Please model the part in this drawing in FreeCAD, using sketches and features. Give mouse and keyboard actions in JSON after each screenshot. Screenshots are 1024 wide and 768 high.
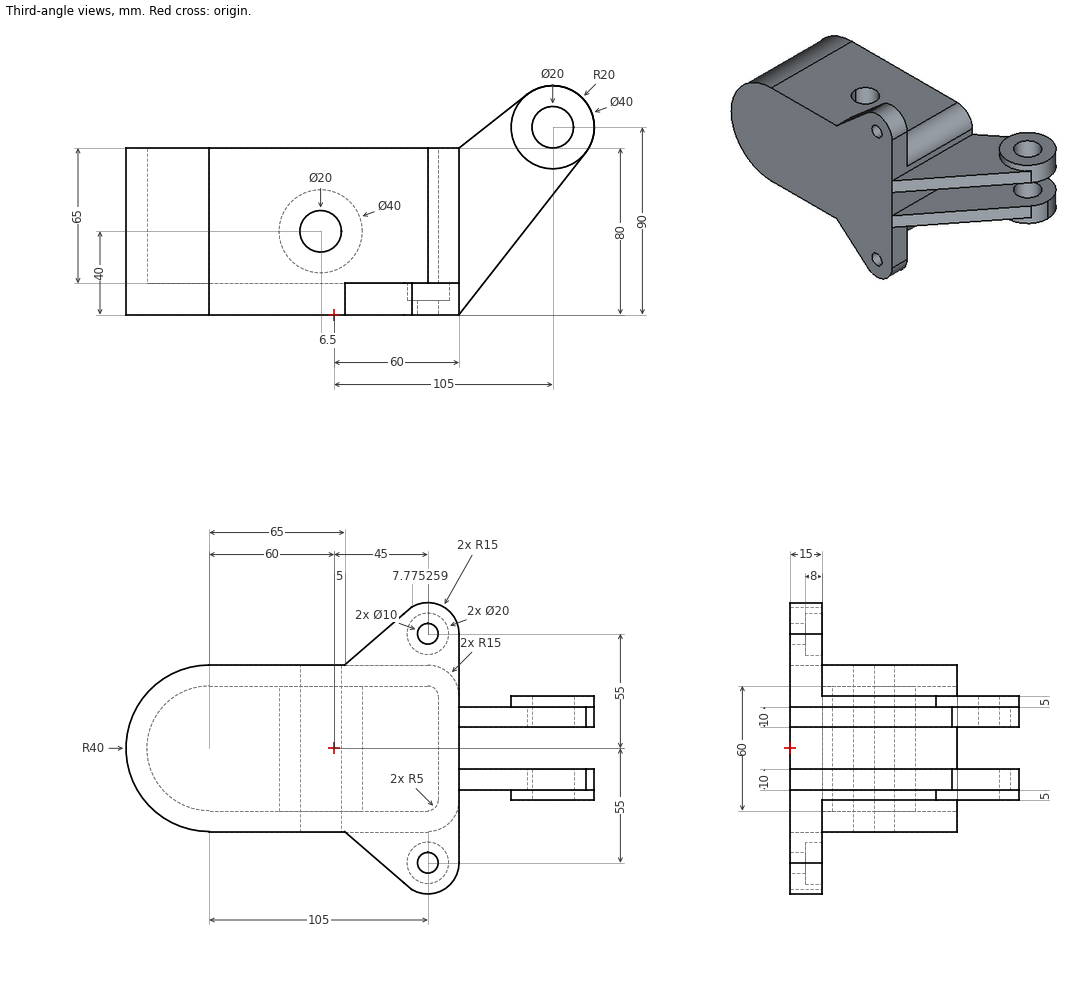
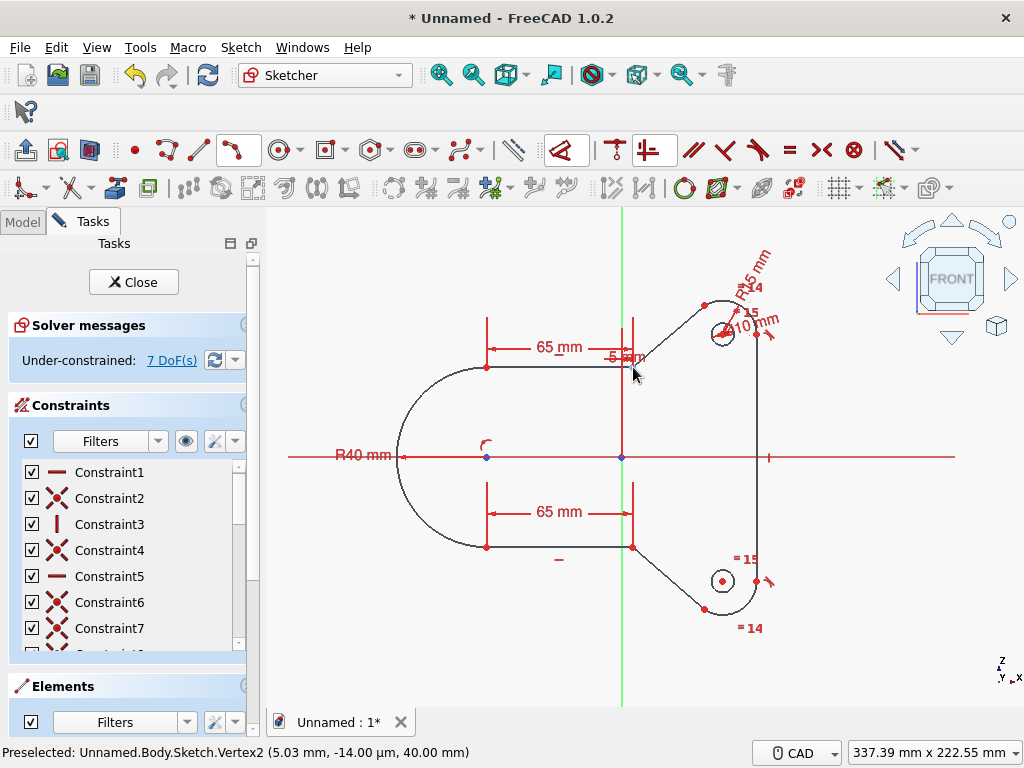
{"action": "scroll", "coordinate": [633, 547], "scroll_direction": "up", "scroll_amount": 7}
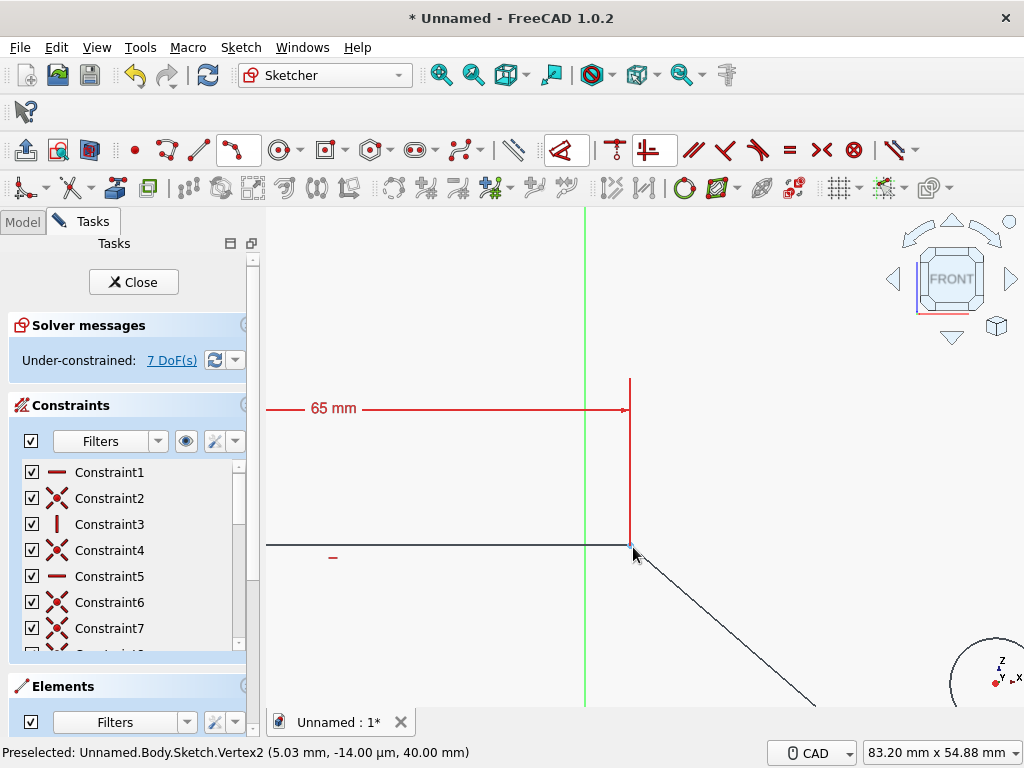
{"action": "left_click", "coordinate": [630, 545]}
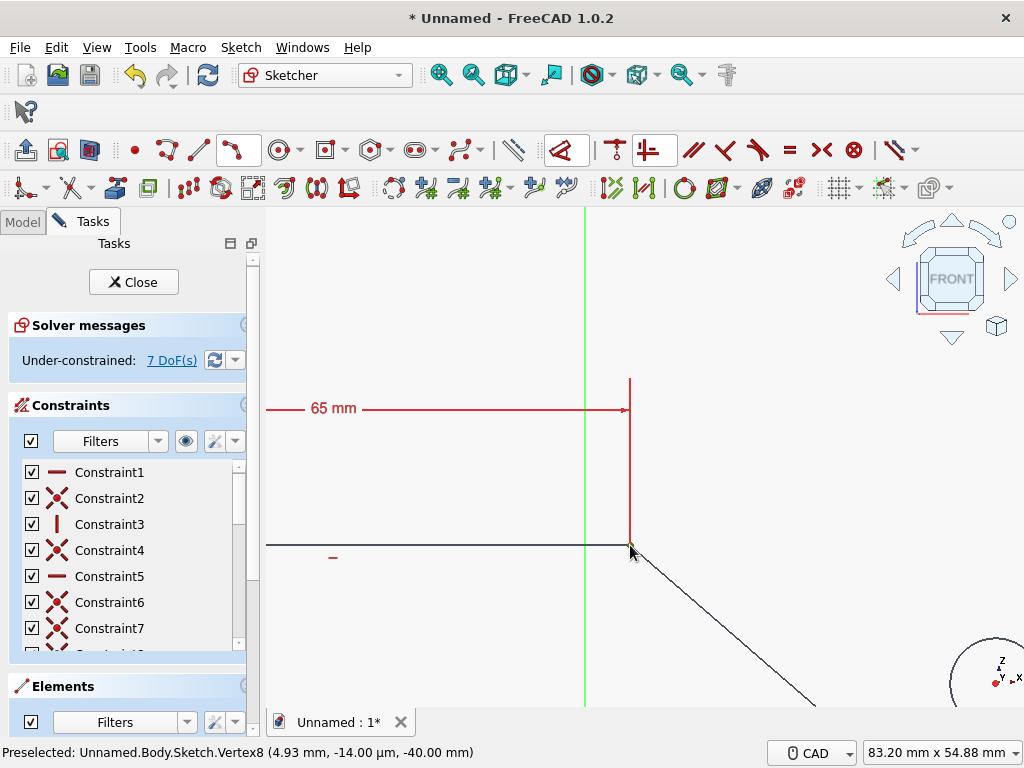
{"action": "key", "text": "l"}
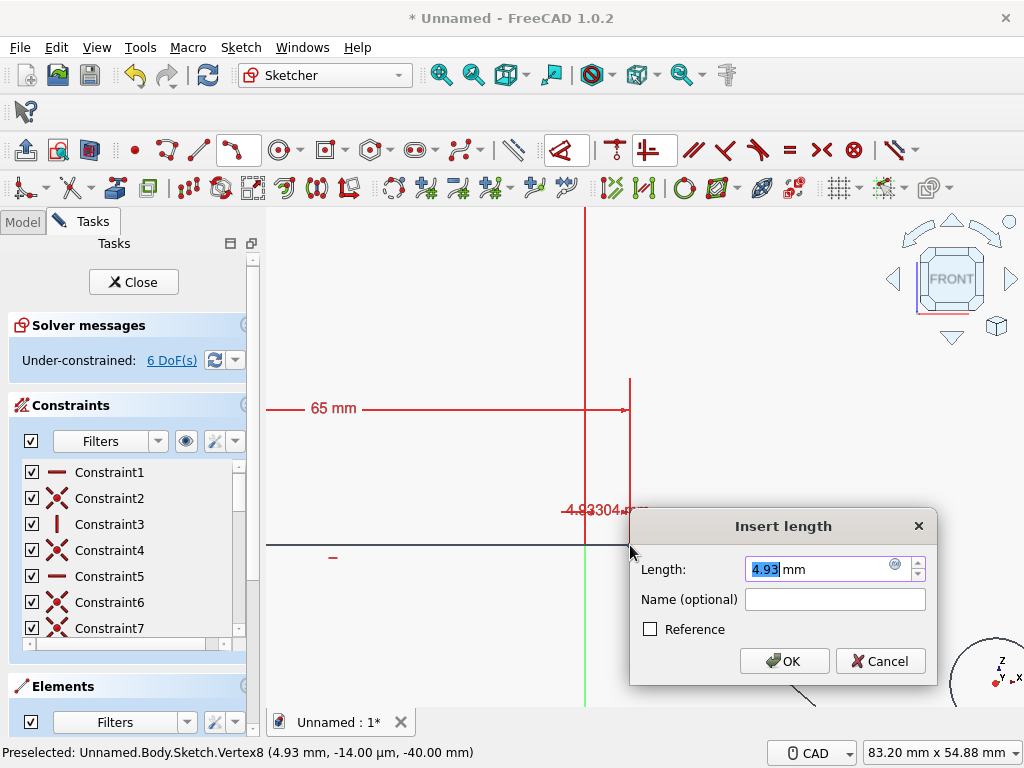
{"action": "type", "text": "5"}
{"action": "key", "text": "Return"}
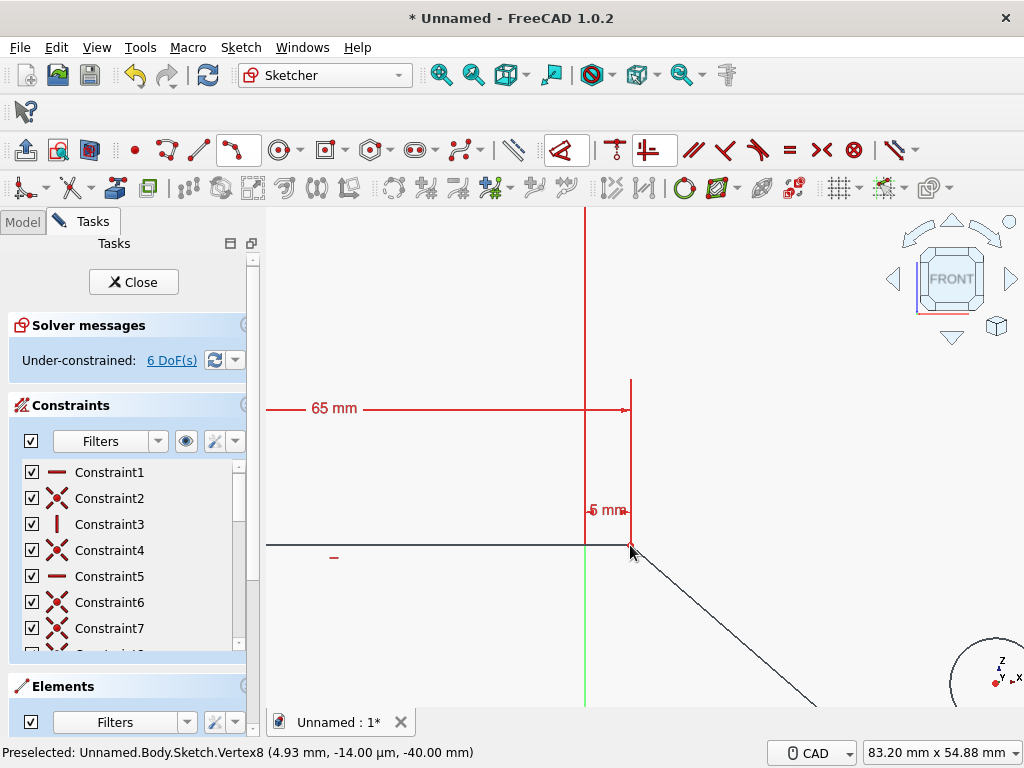
{"action": "scroll", "coordinate": [633, 547], "scroll_direction": "down", "scroll_amount": 7}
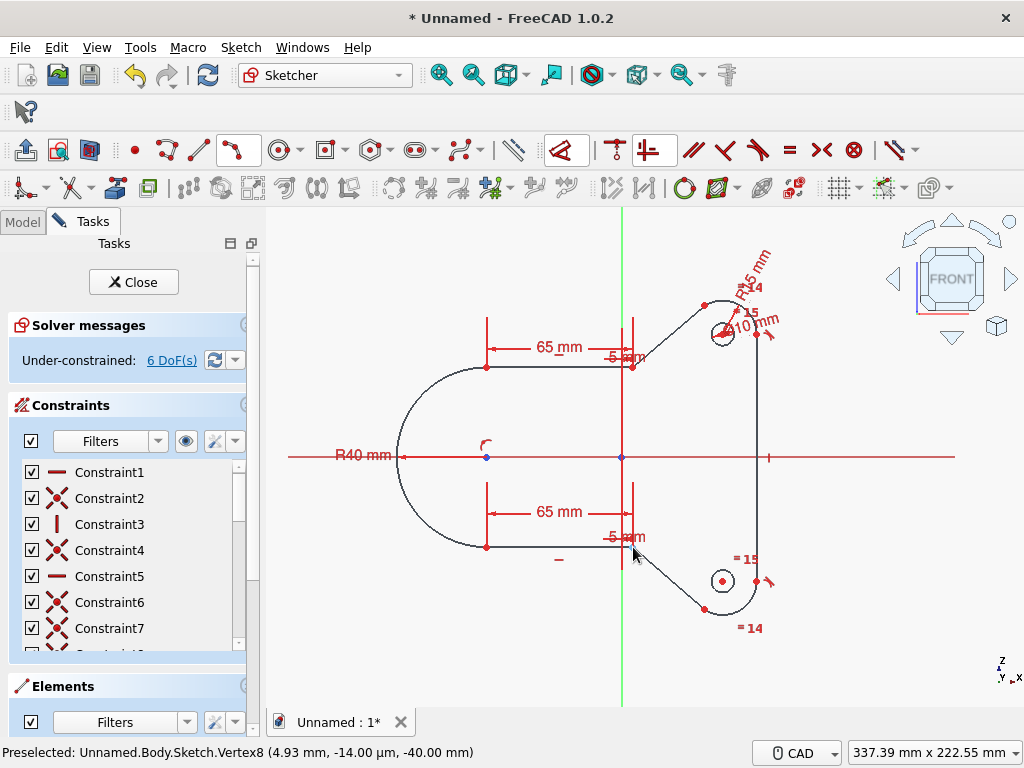
{"action": "left_click", "coordinate": [723, 334]}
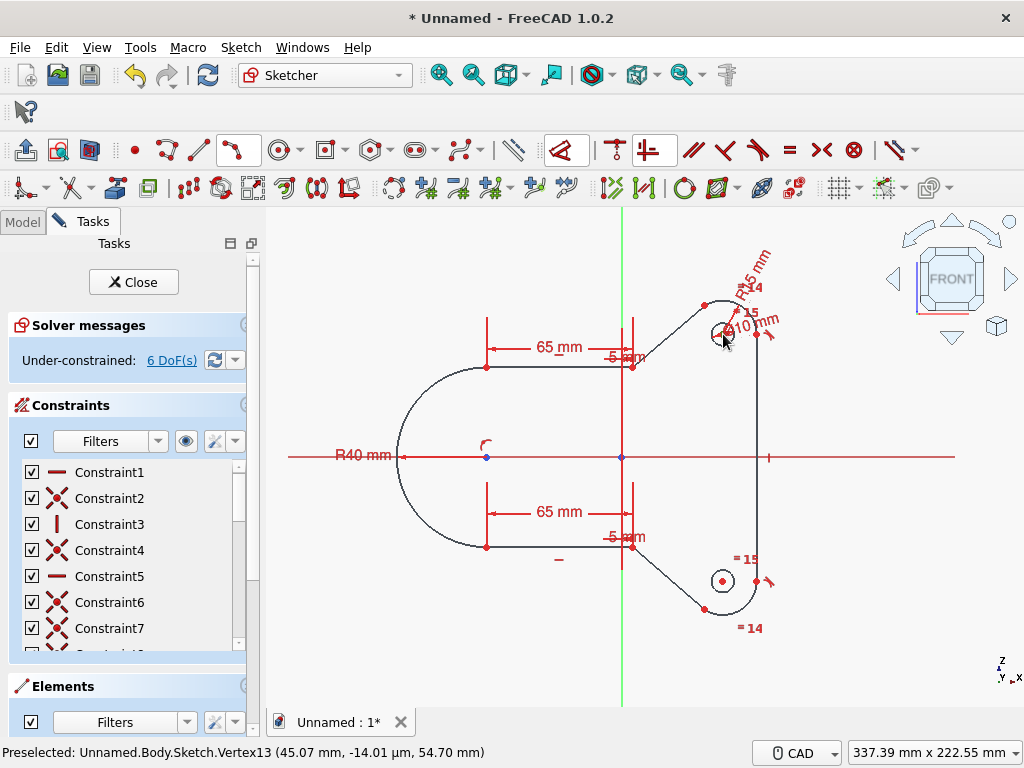
{"action": "left_click", "coordinate": [584, 150]}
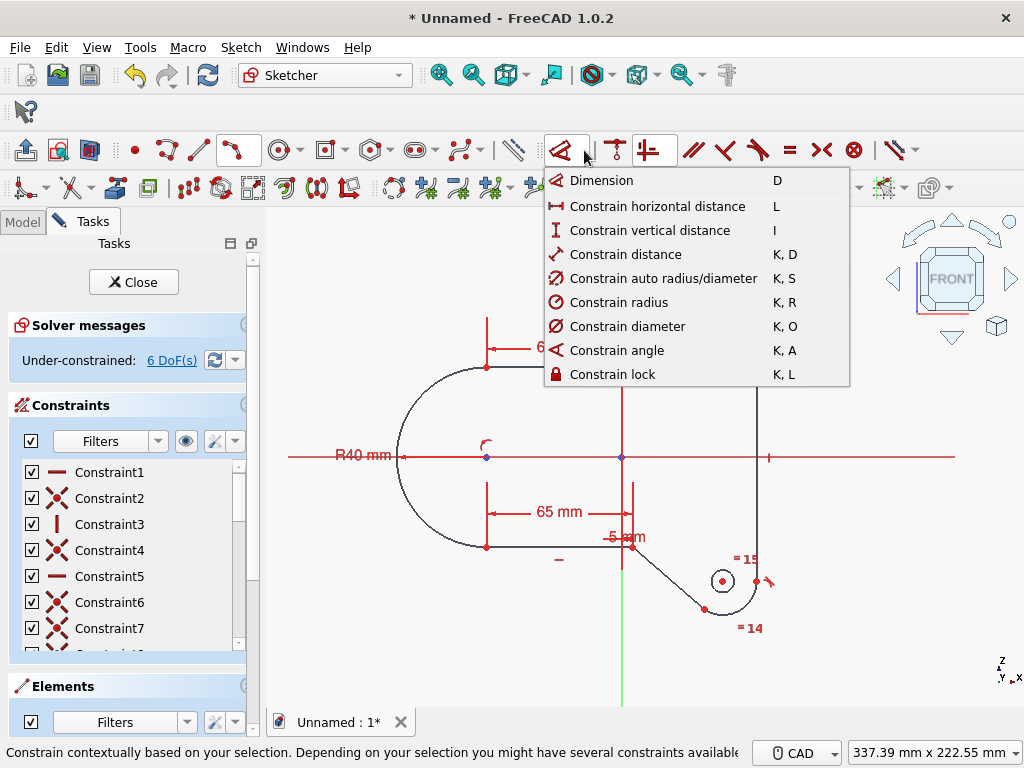
{"action": "left_click", "coordinate": [697, 206]}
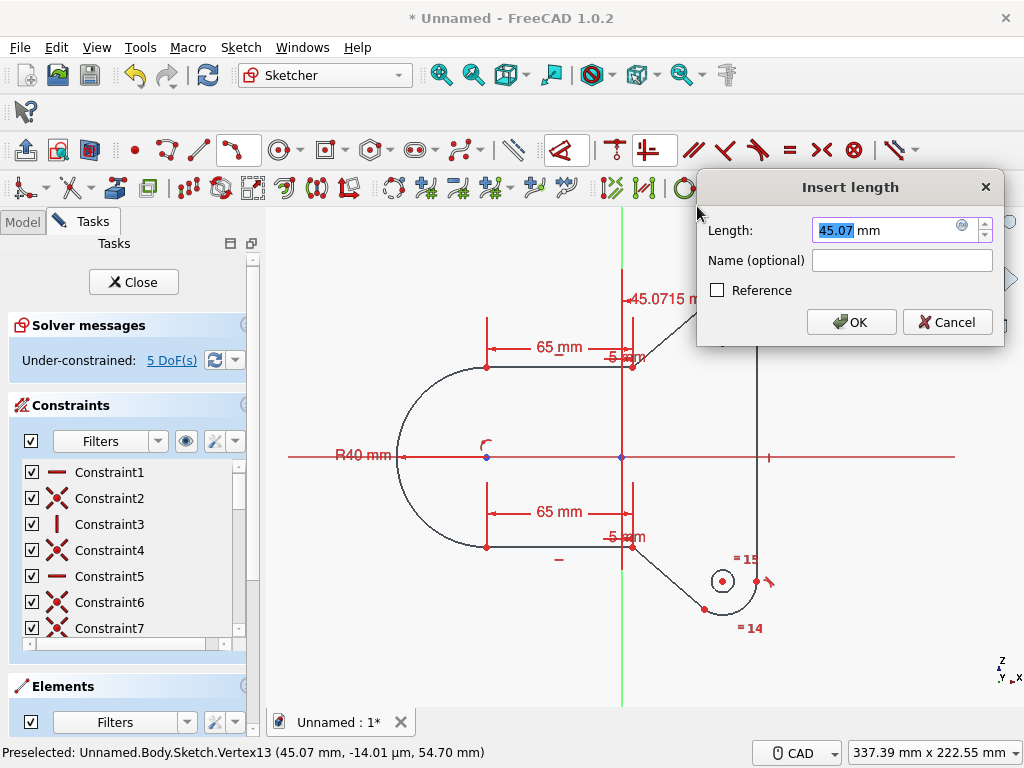
{"action": "type", "text": "45"}
{"action": "key", "text": "Return"}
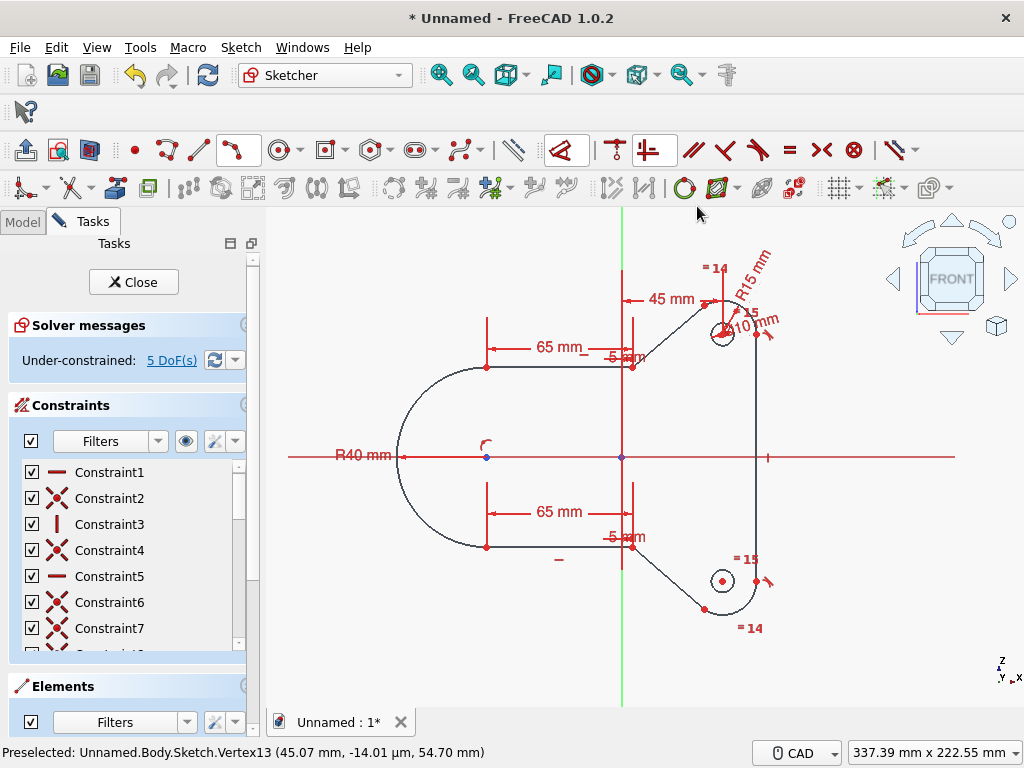
{"action": "left_click", "coordinate": [723, 334]}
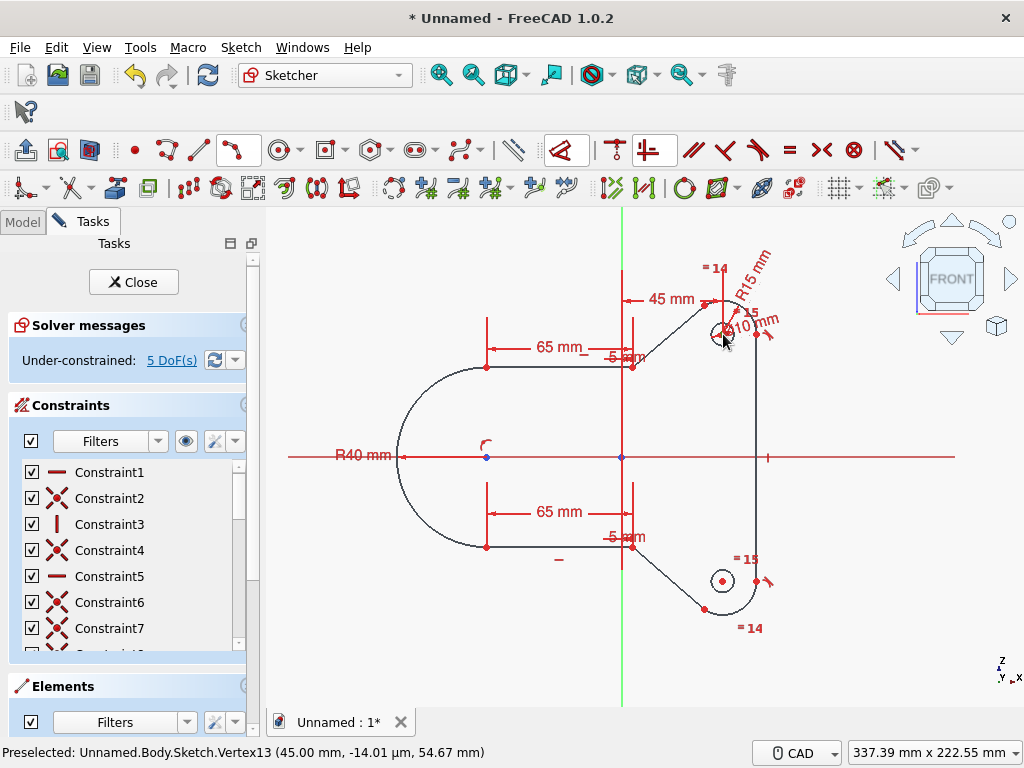
{"action": "left_click", "coordinate": [584, 150]}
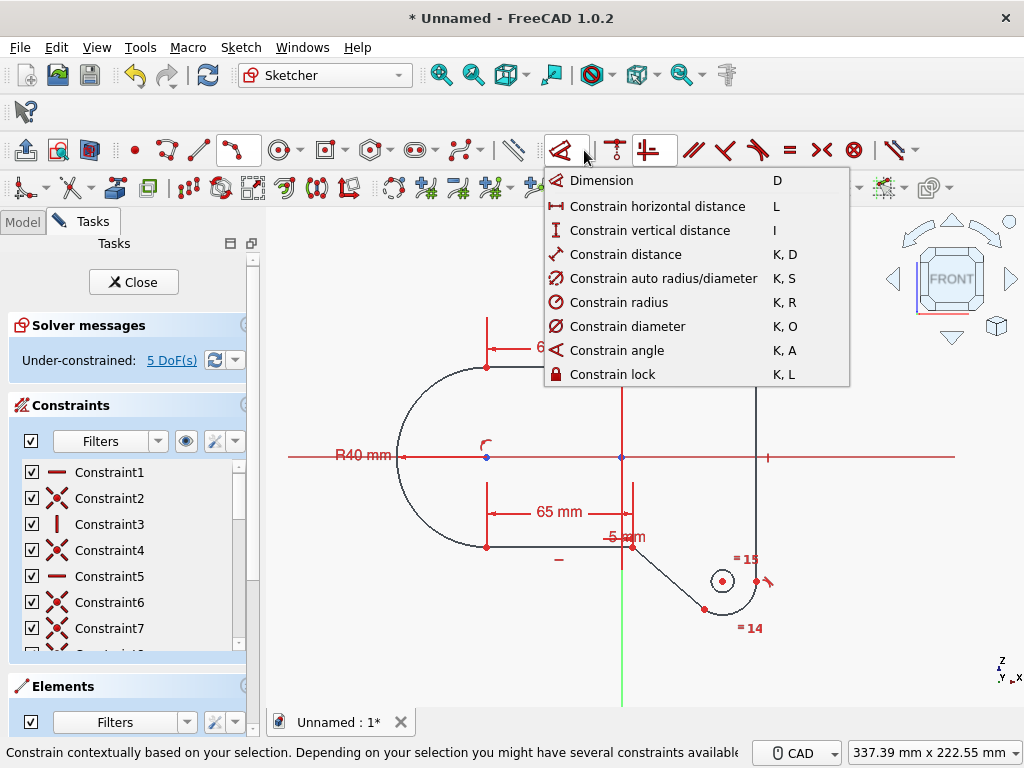
{"action": "left_click", "coordinate": [697, 230]}